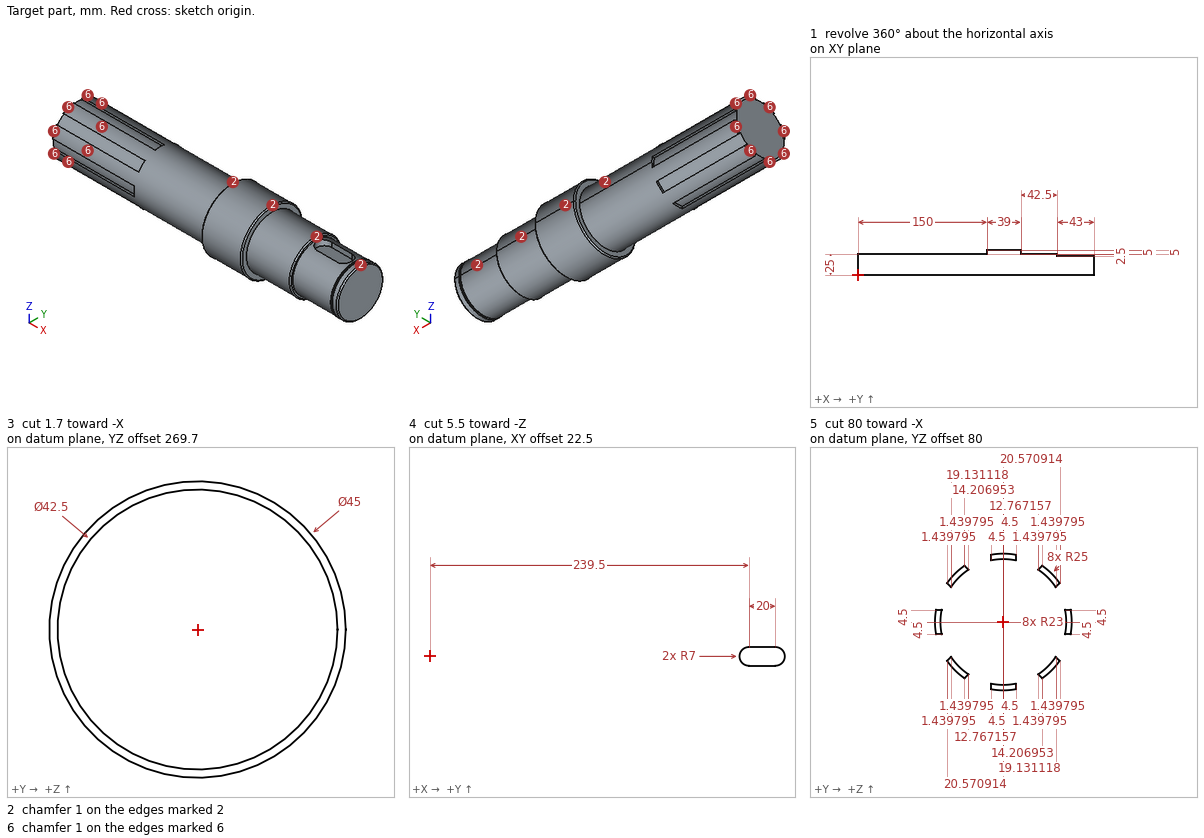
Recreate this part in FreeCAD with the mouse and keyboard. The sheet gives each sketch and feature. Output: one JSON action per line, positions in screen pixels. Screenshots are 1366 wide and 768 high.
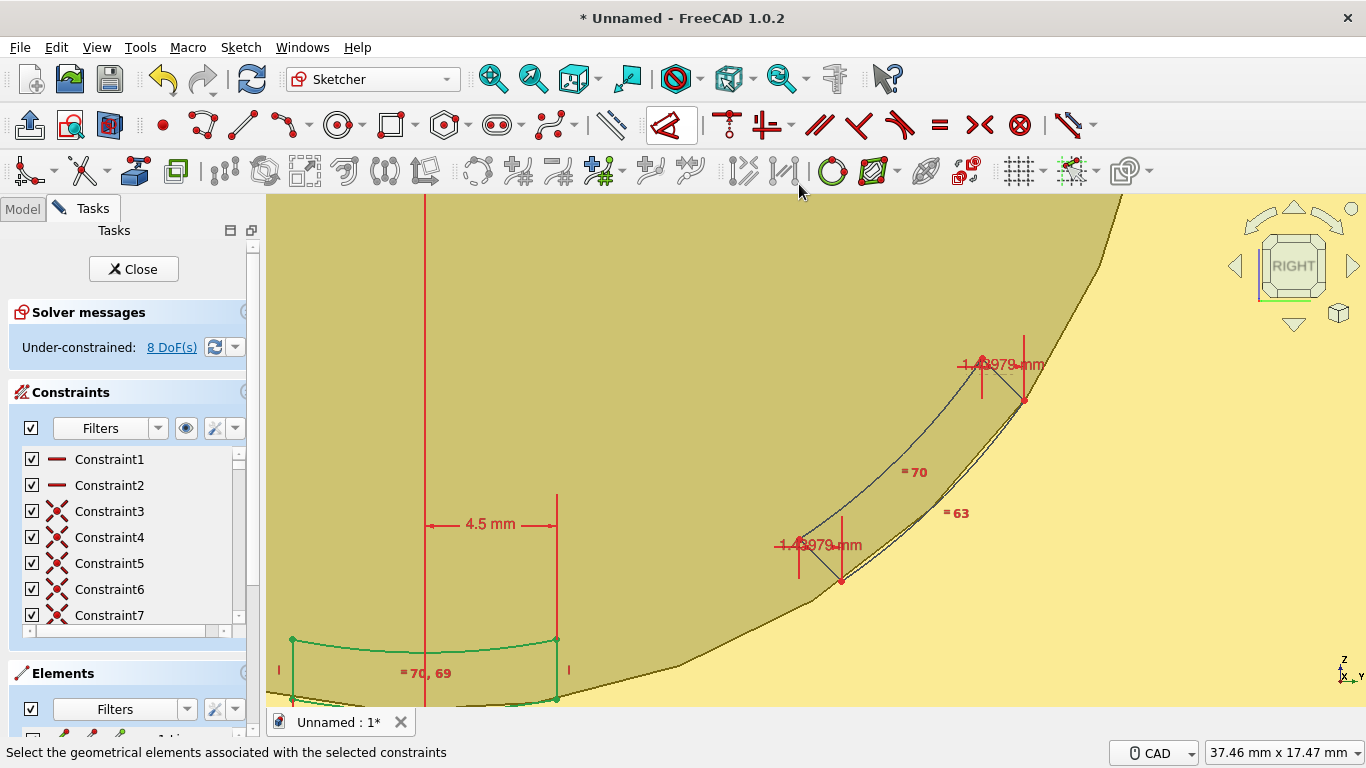
{"action": "scroll", "coordinate": [829, 570], "scroll_direction": "down", "scroll_amount": 8}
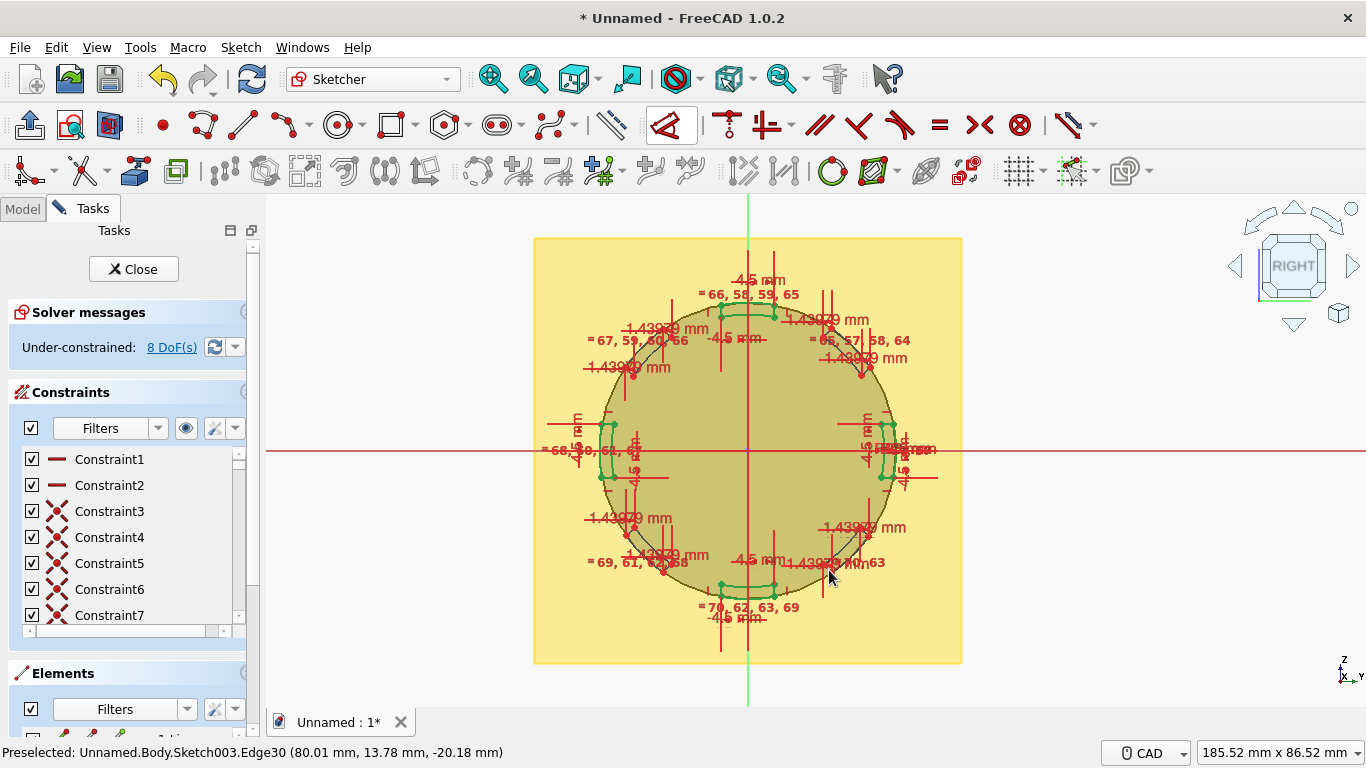
{"action": "left_click", "coordinate": [823, 337]}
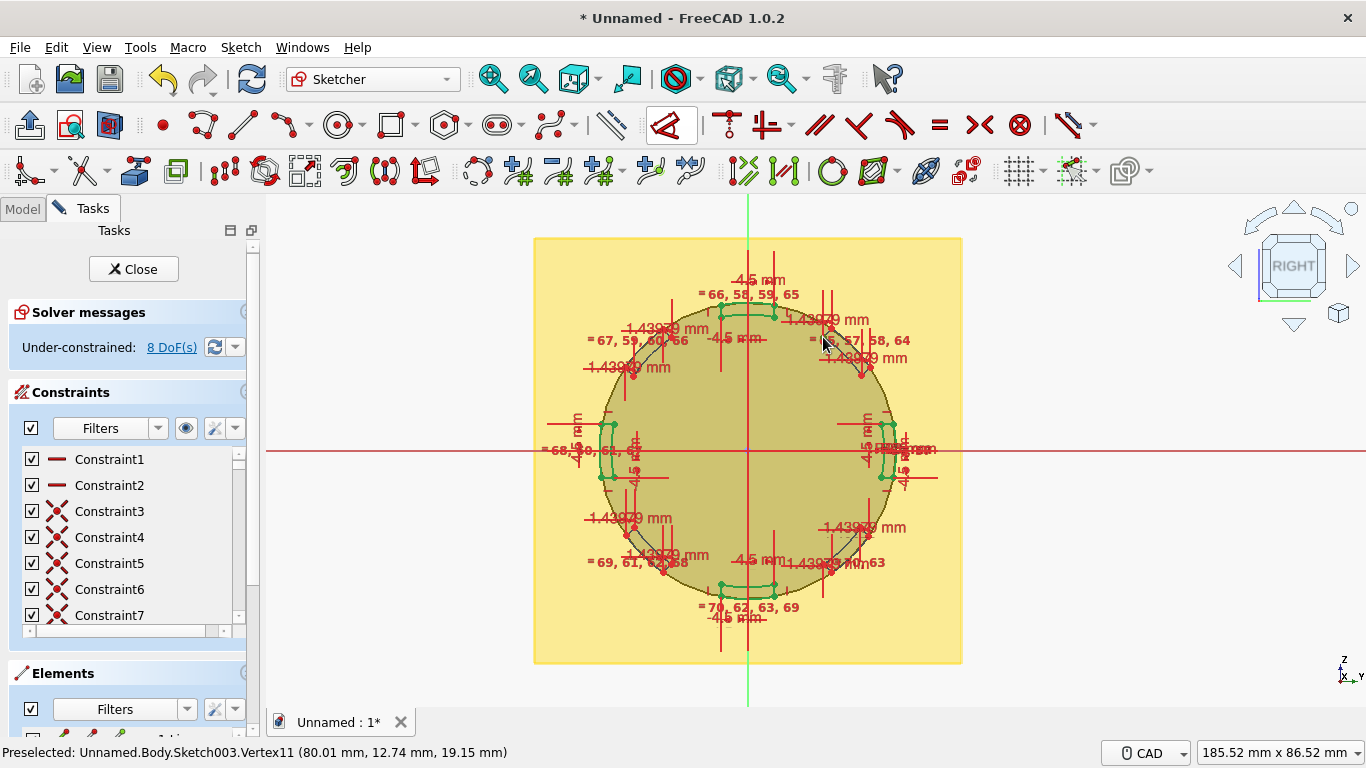
{"action": "left_click", "coordinate": [692, 126]}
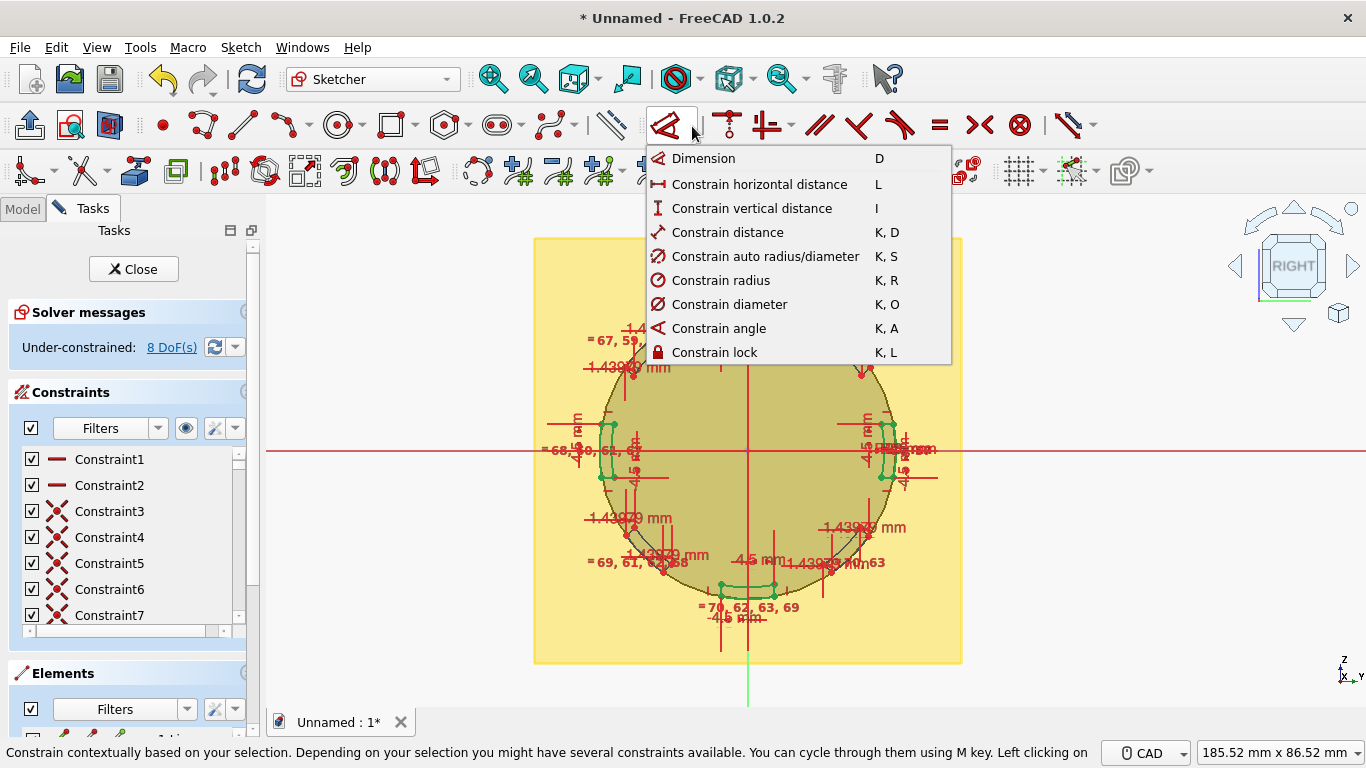
{"action": "left_click", "coordinate": [799, 184]}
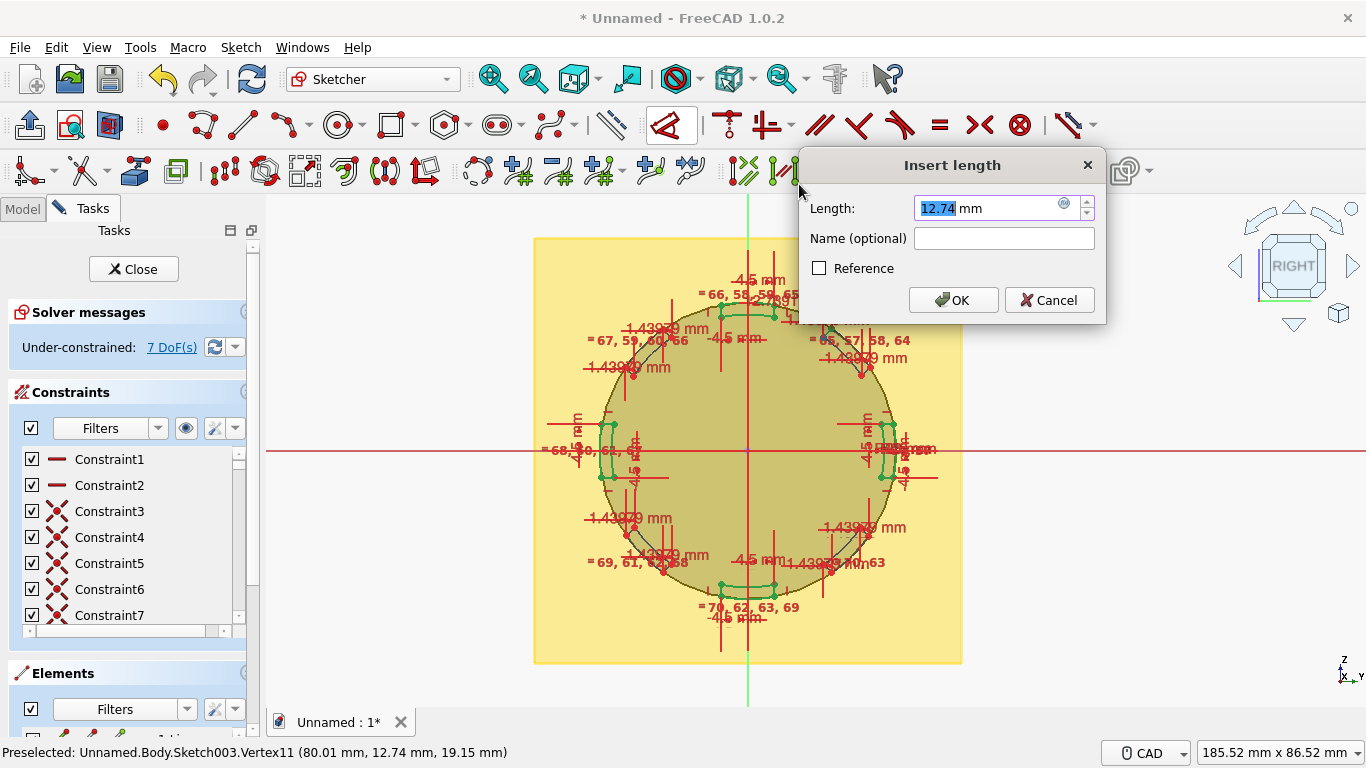
{"action": "type", "text": "12.767157"}
{"action": "key", "text": "Return"}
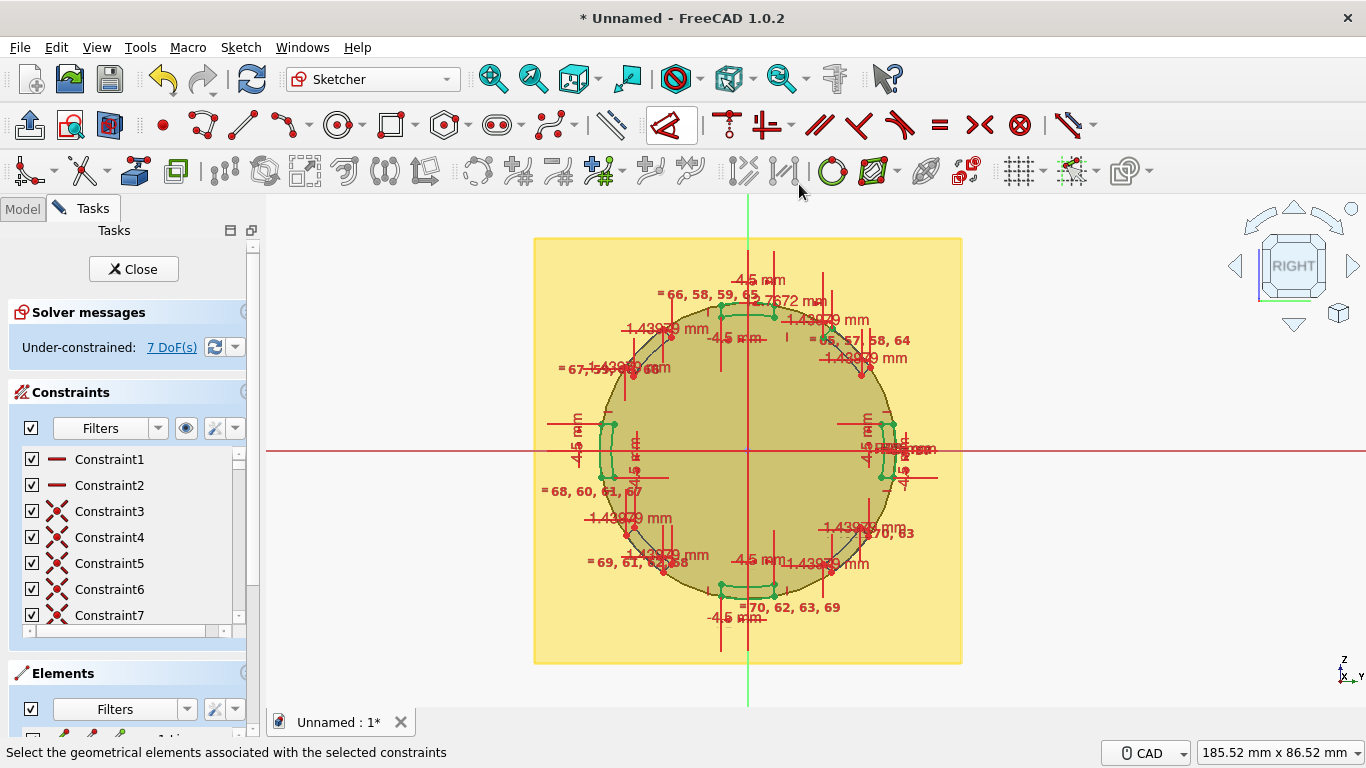
{"action": "left_click", "coordinate": [870, 367]}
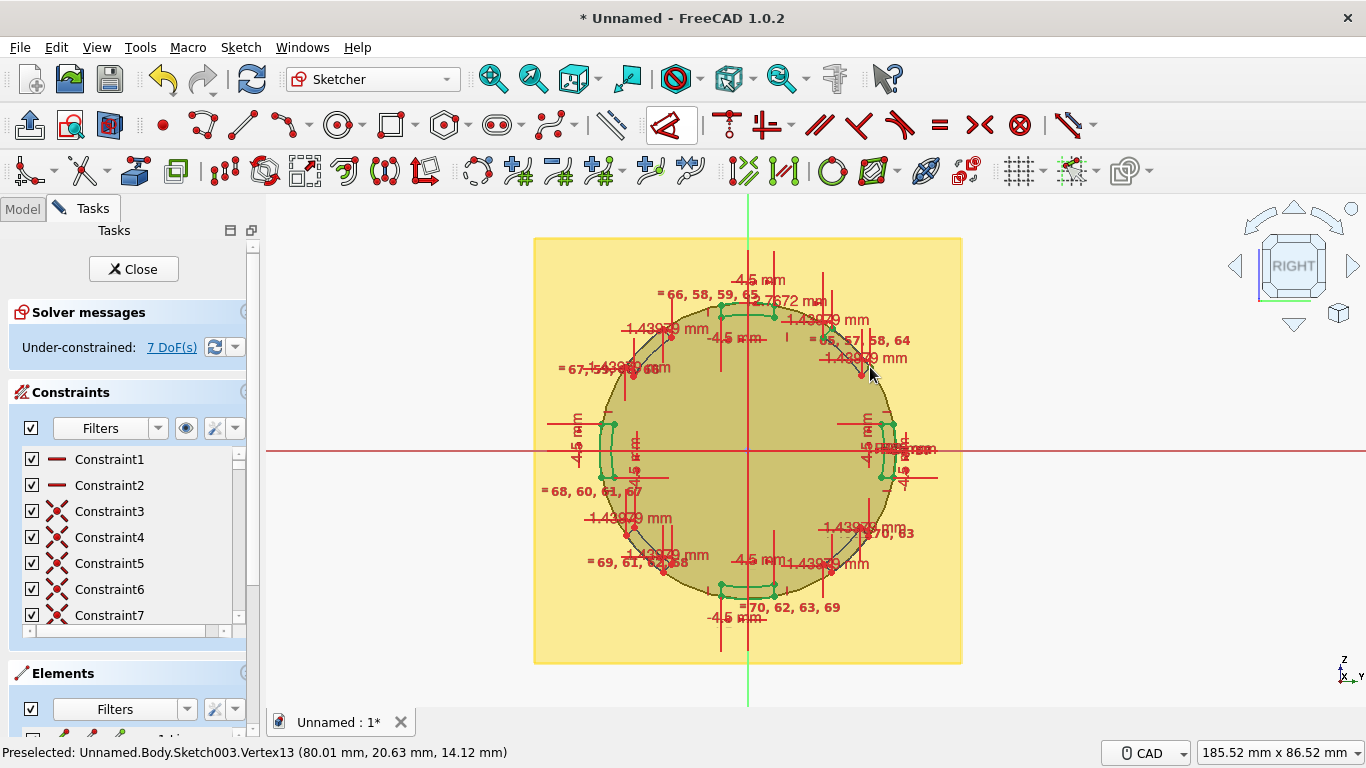
{"action": "key", "text": "l"}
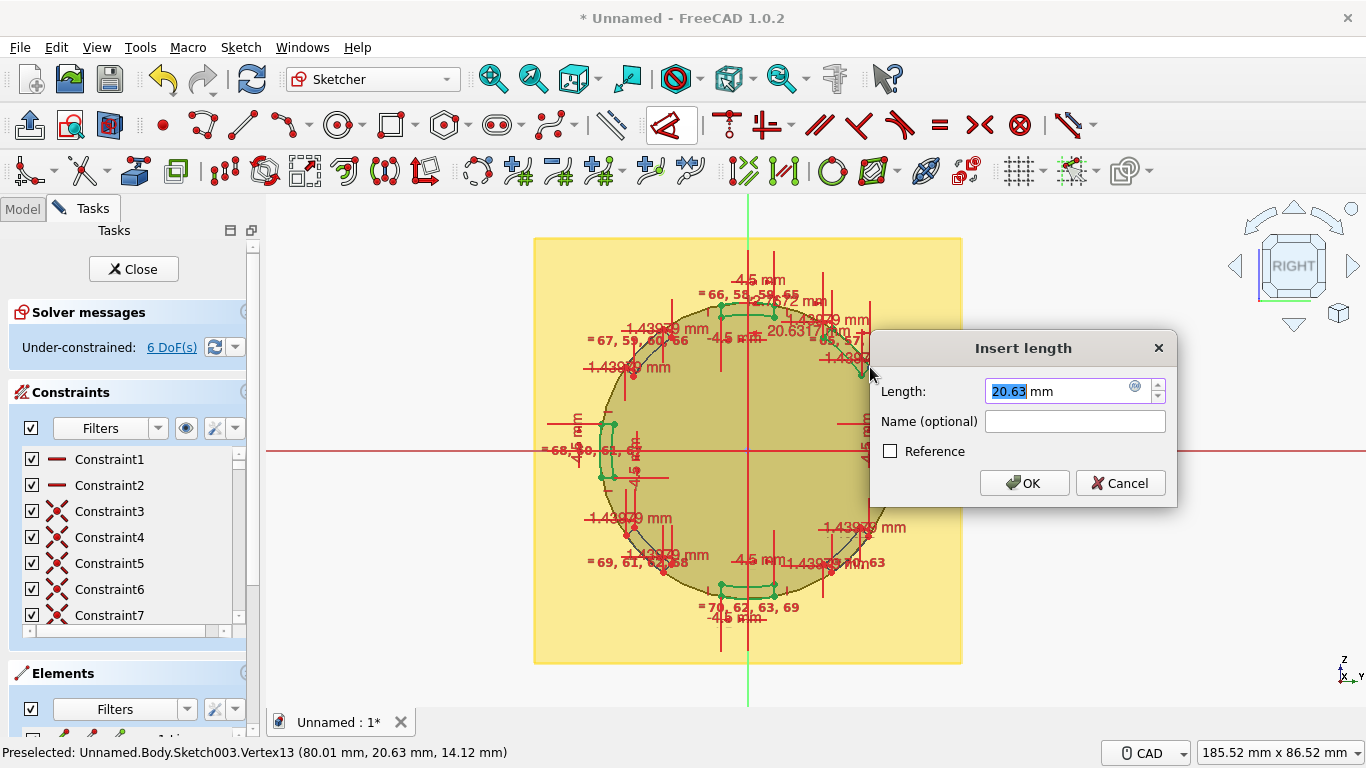
{"action": "type", "text": "20.570914"}
{"action": "key", "text": "Return"}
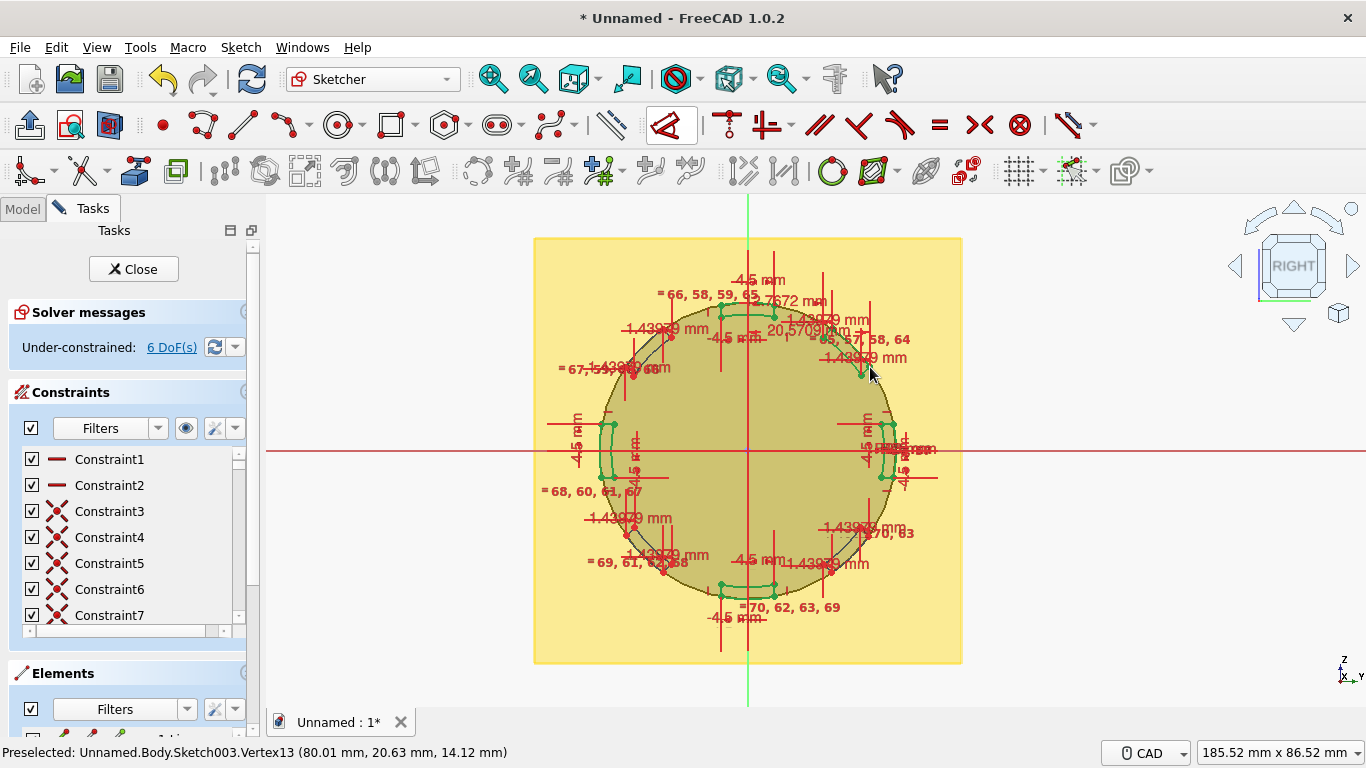
{"action": "left_click", "coordinate": [634, 376]}